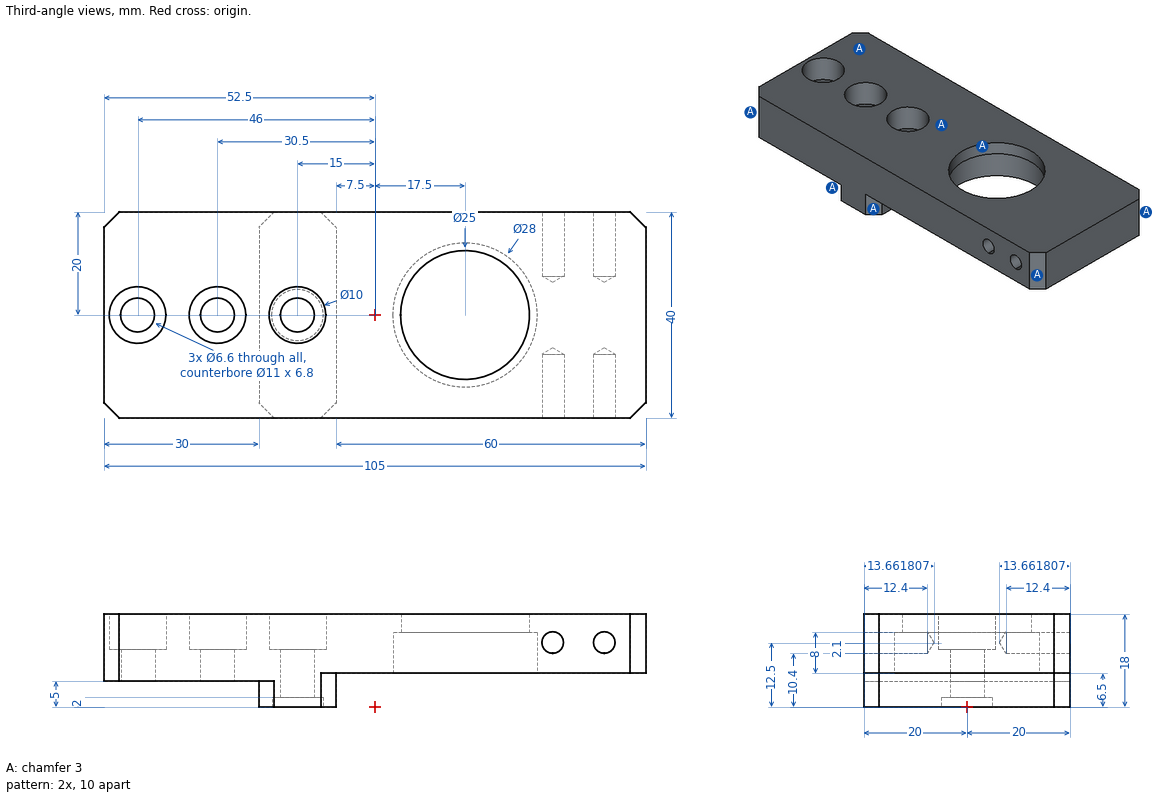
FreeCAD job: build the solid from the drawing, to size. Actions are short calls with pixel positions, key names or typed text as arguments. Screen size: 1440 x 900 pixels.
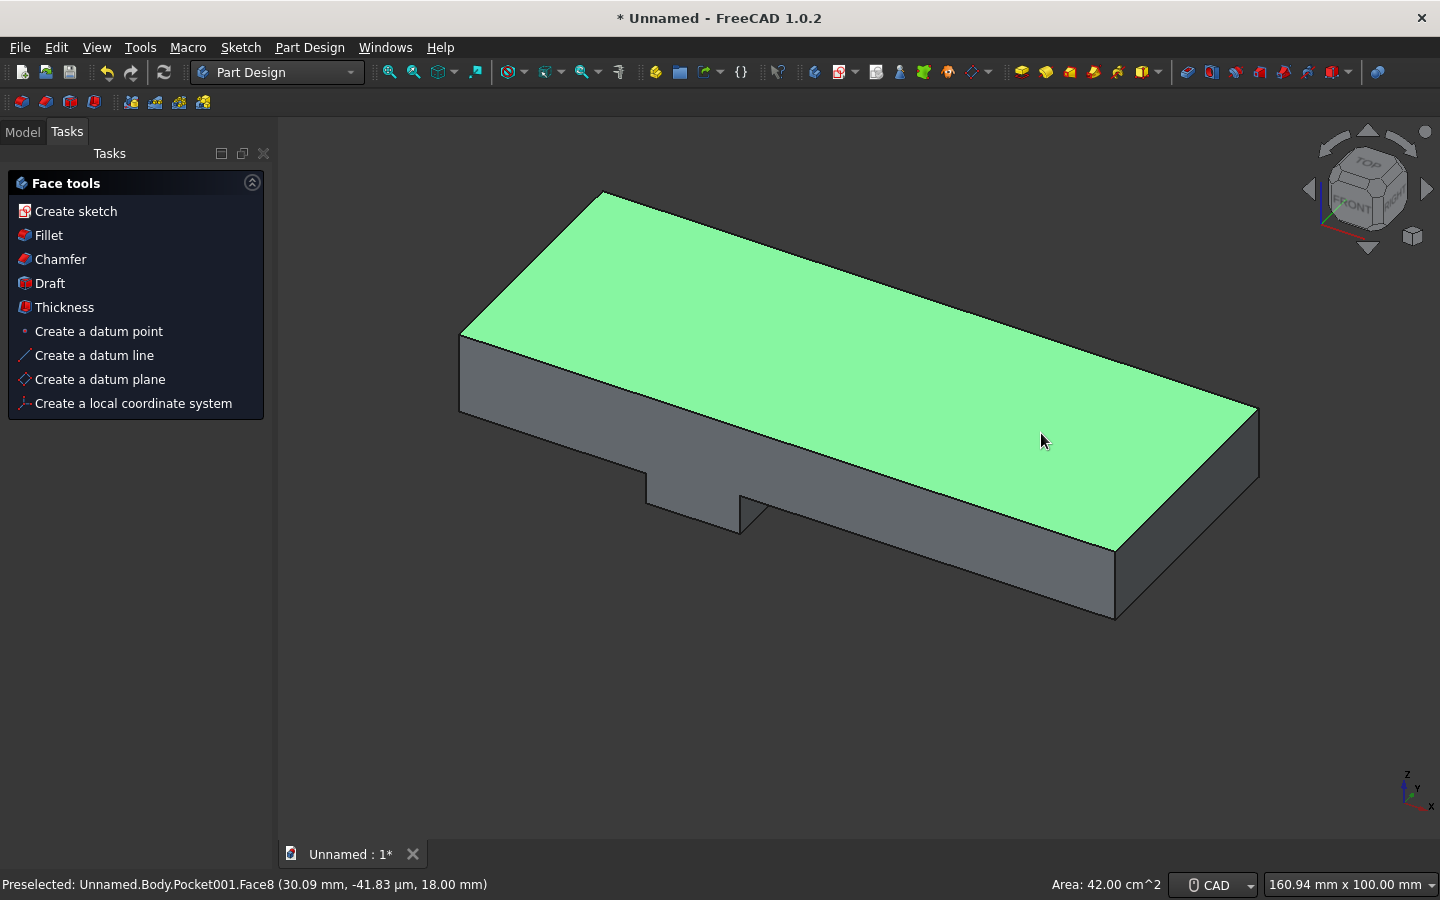
click(840, 72)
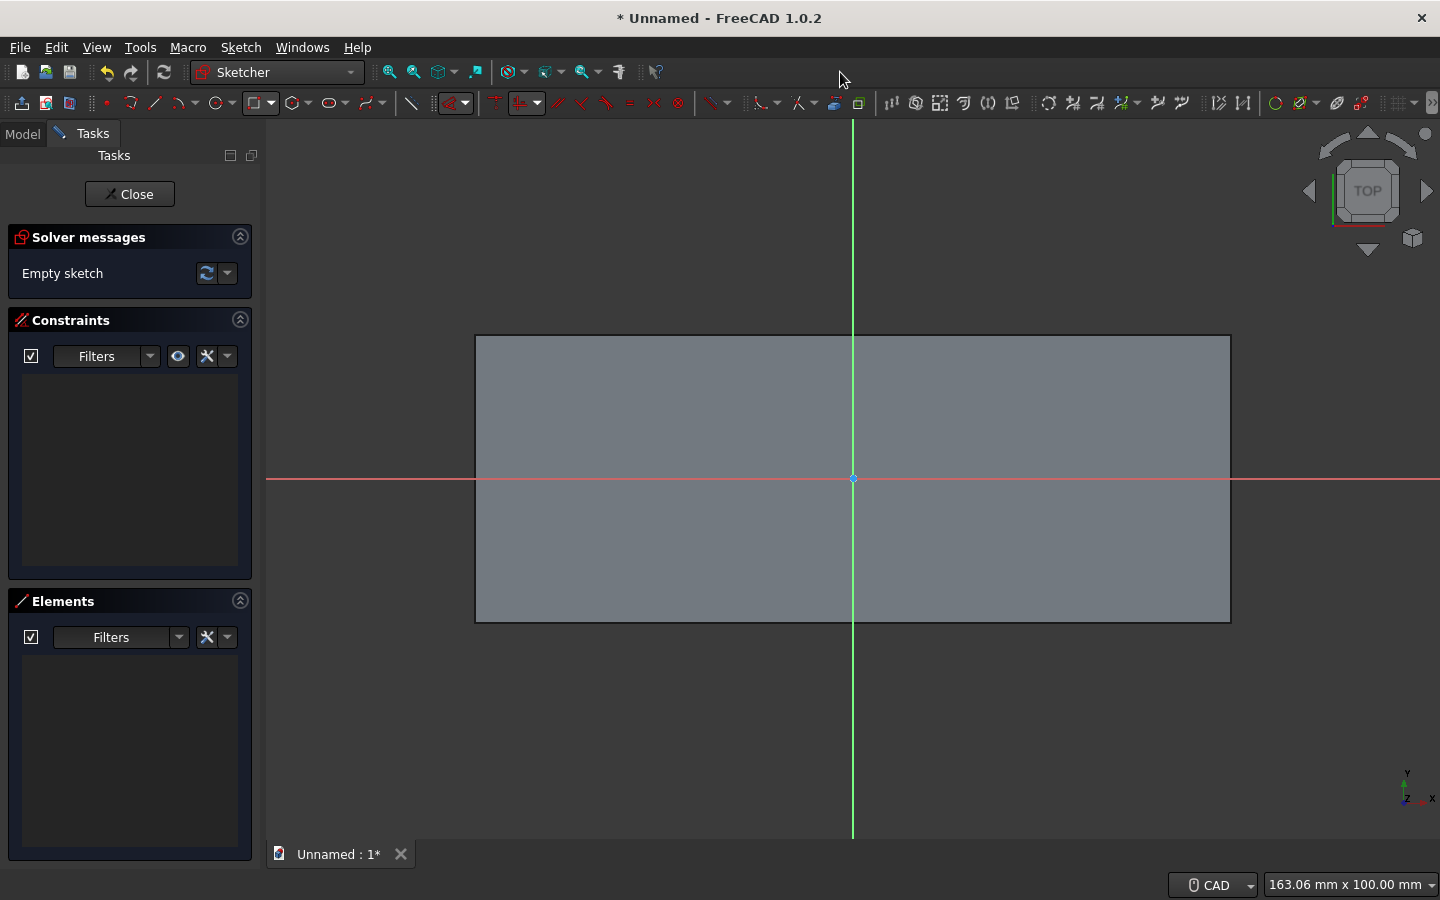
scroll(543, 479, up, 3)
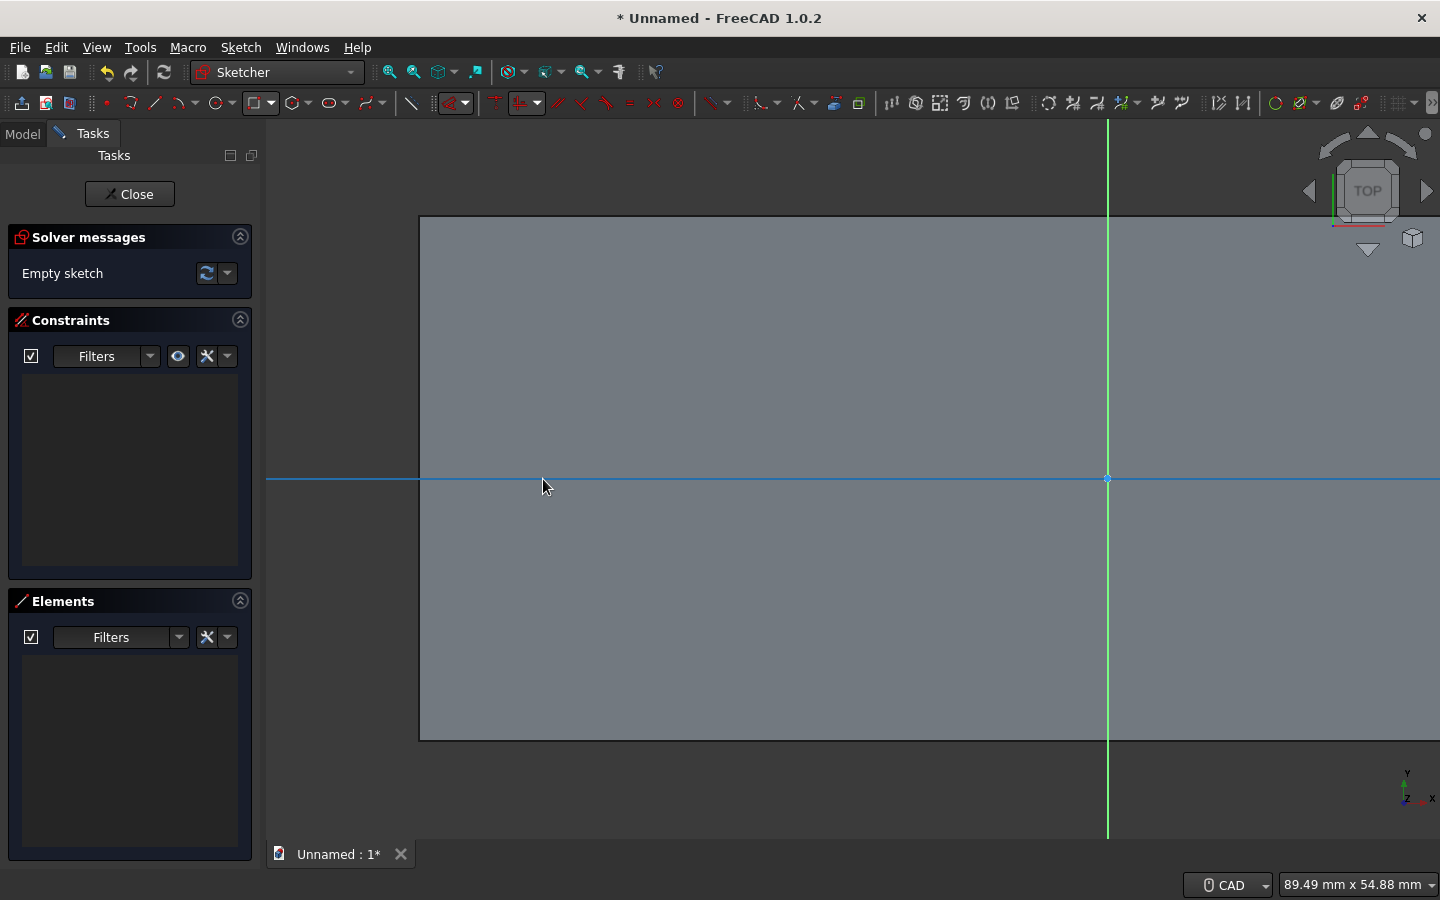
click(216, 104)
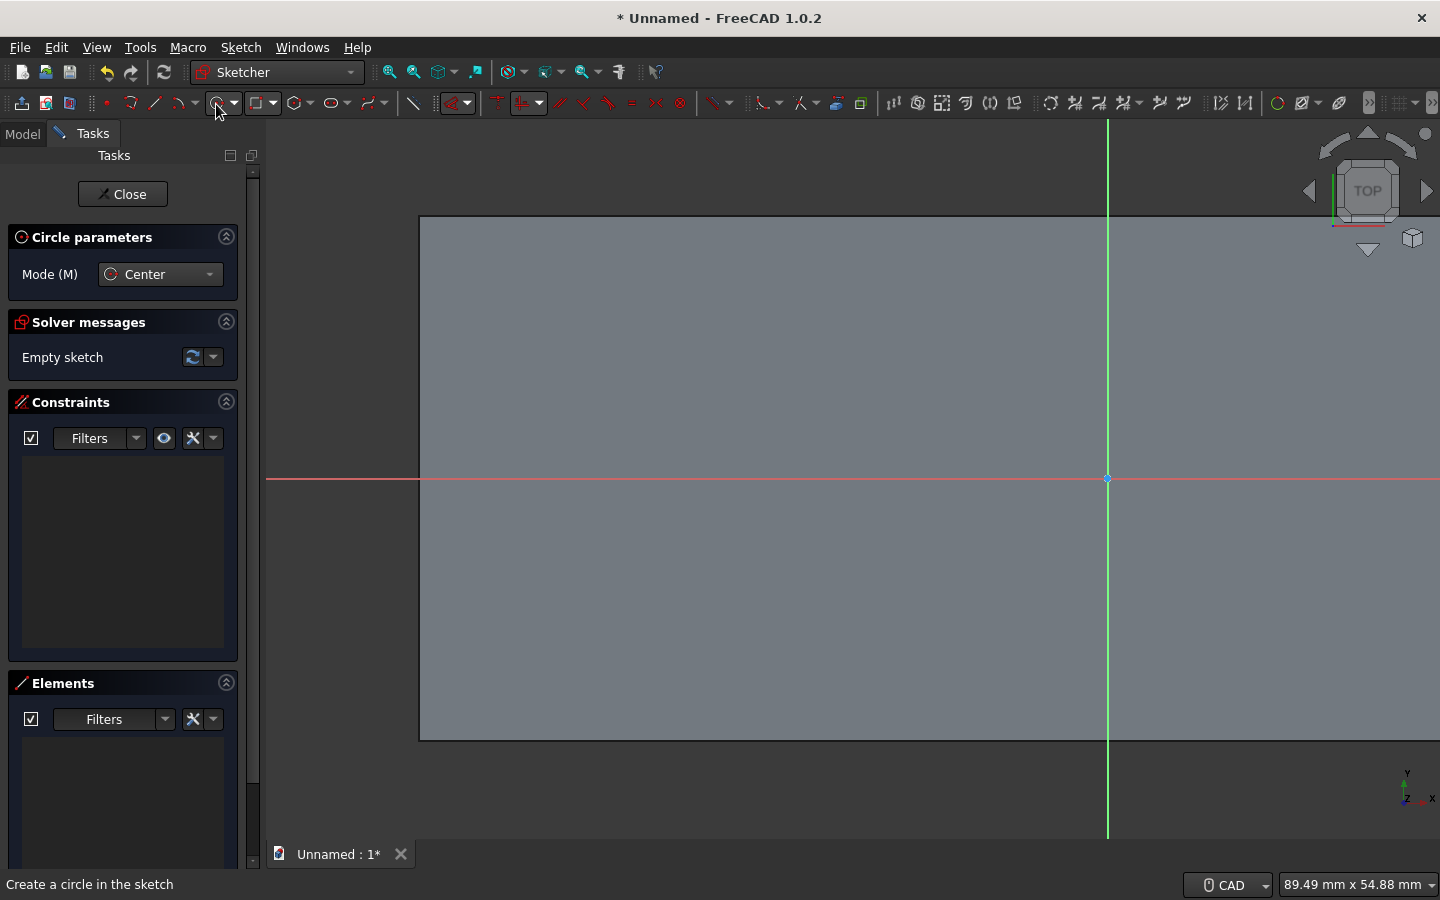
click(504, 479)
click(535, 448)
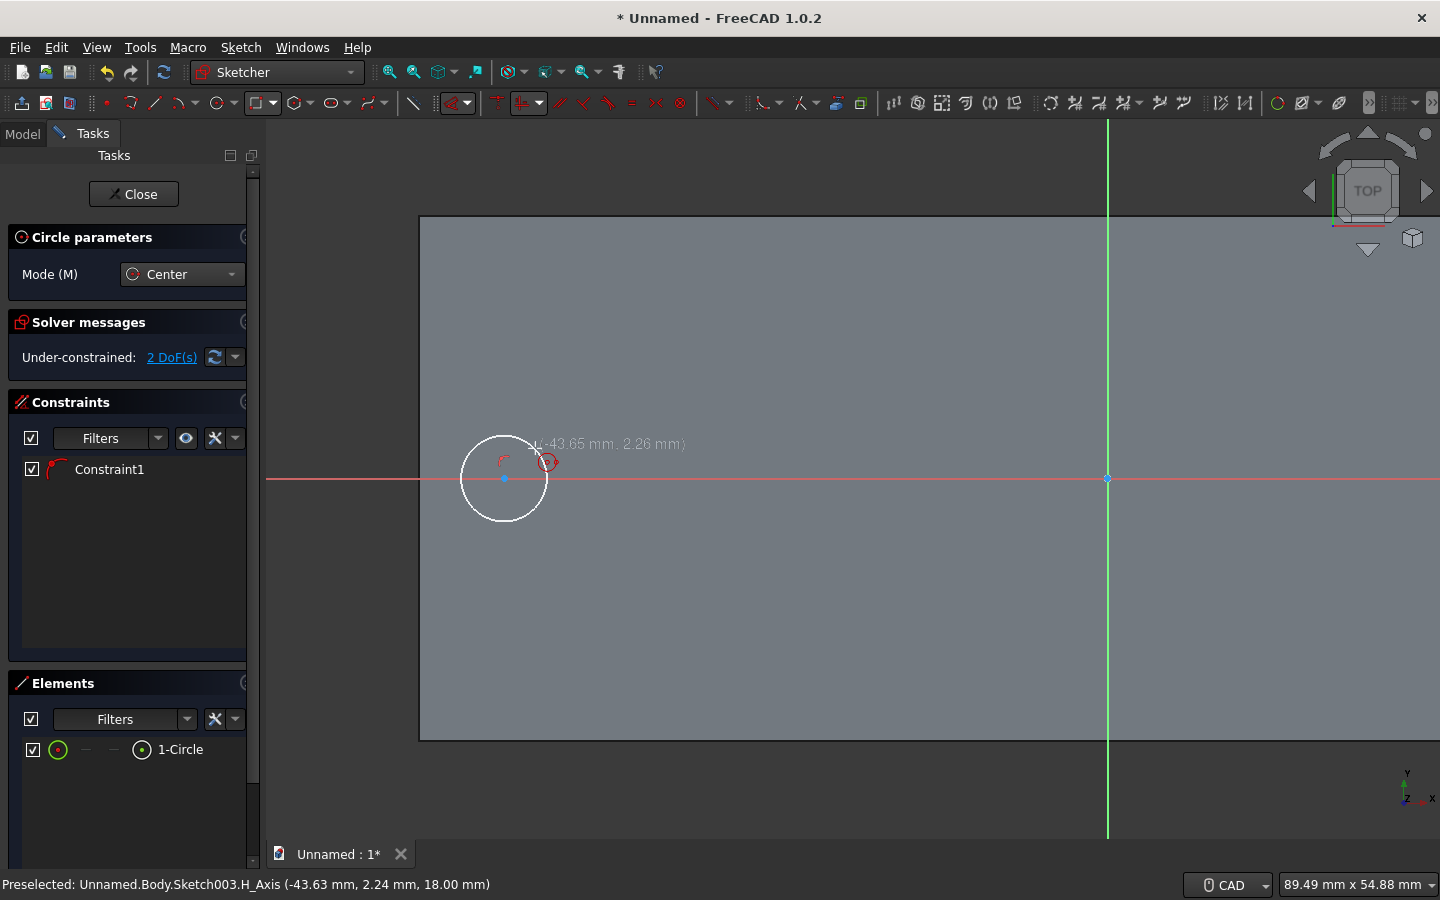
click(708, 479)
click(738, 448)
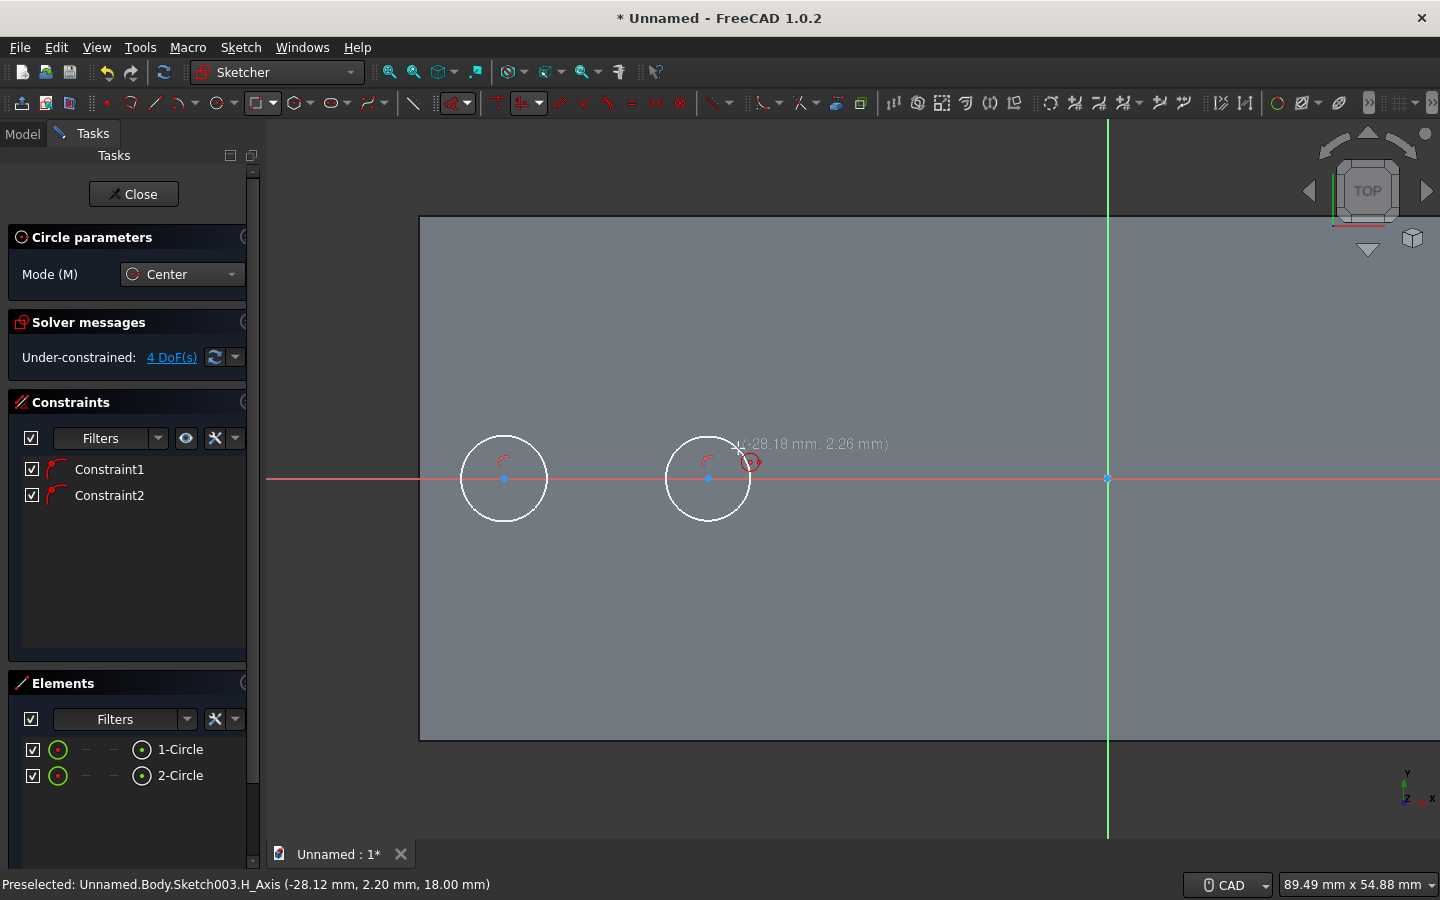
click(911, 479)
click(941, 448)
key(Escape)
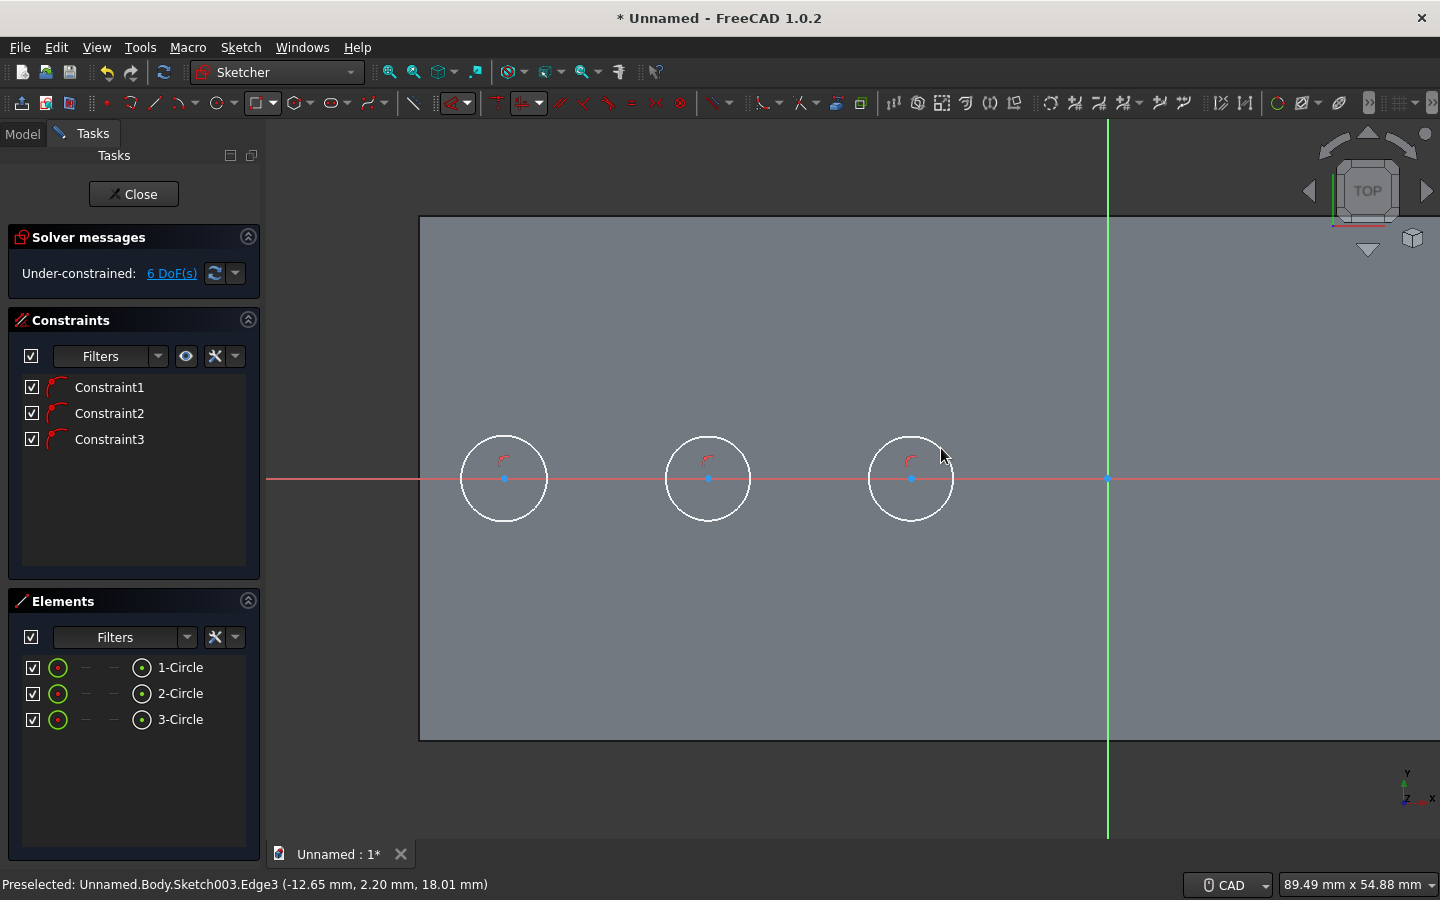
click(534, 448)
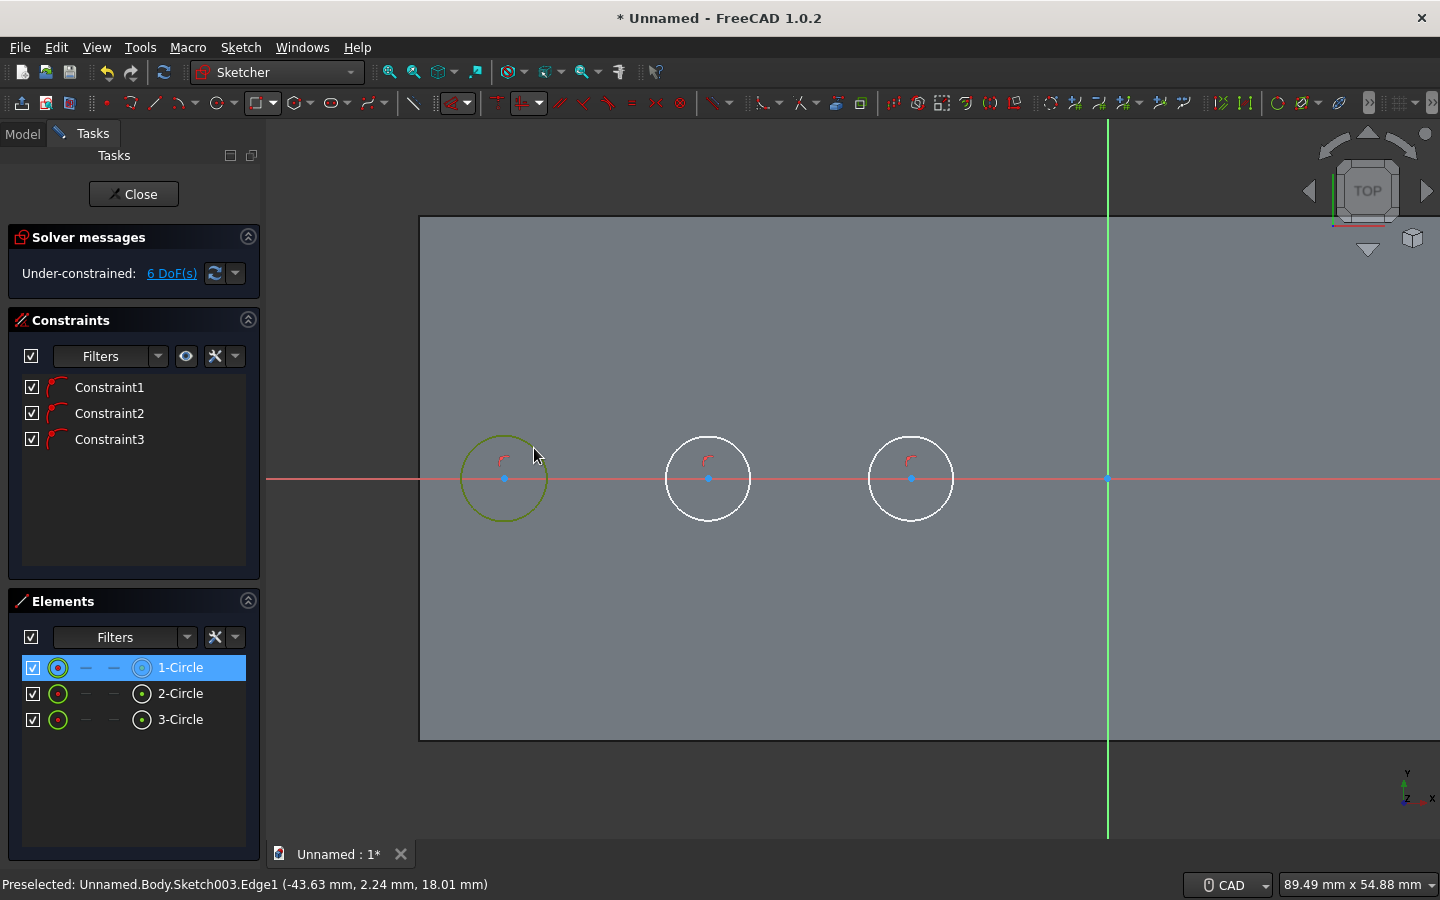
click(738, 449)